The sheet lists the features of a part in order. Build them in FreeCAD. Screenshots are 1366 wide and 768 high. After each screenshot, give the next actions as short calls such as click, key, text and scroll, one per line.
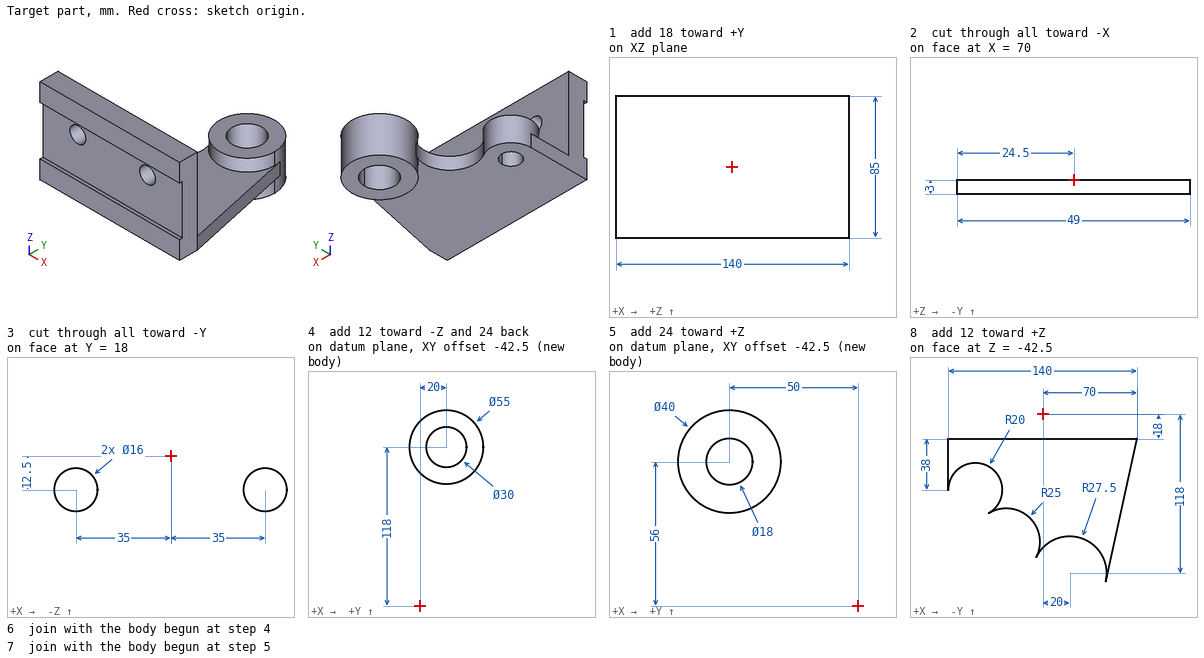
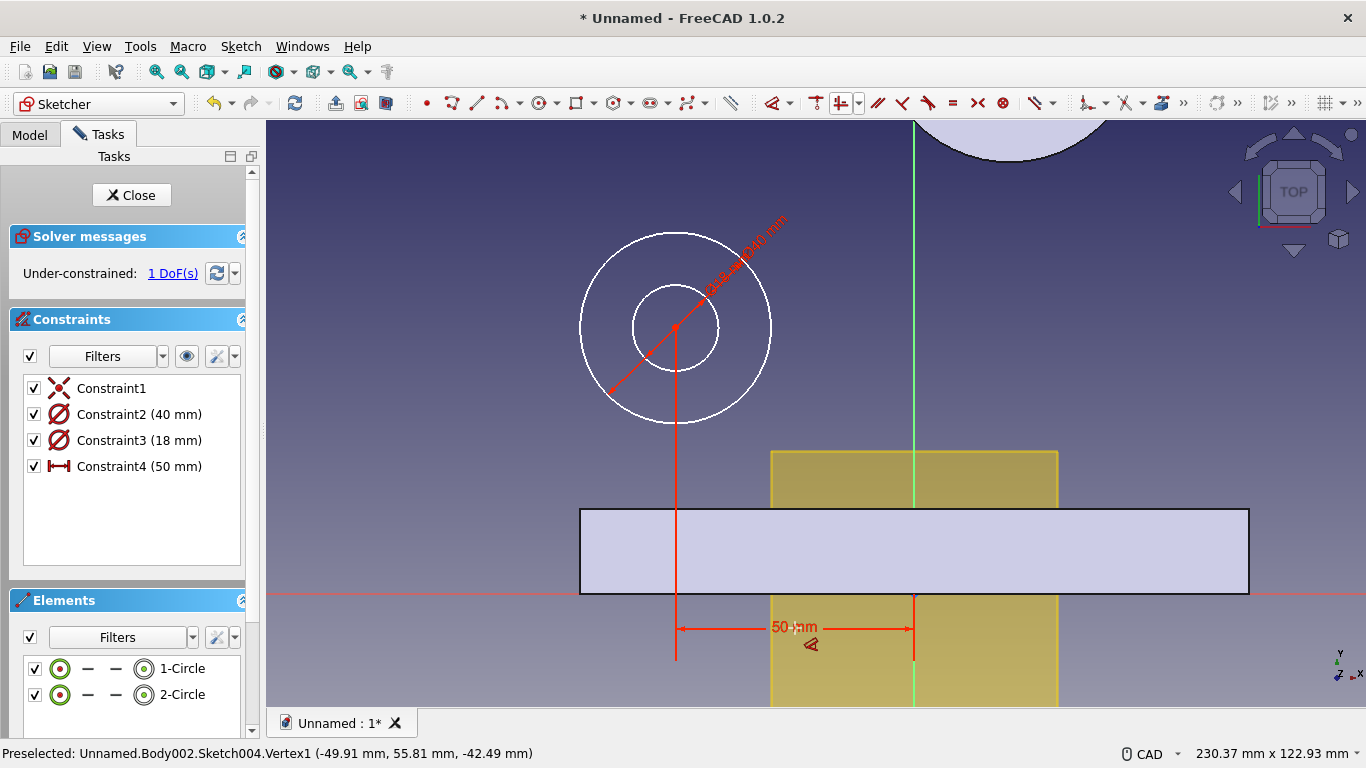
click(676, 328)
click(948, 461)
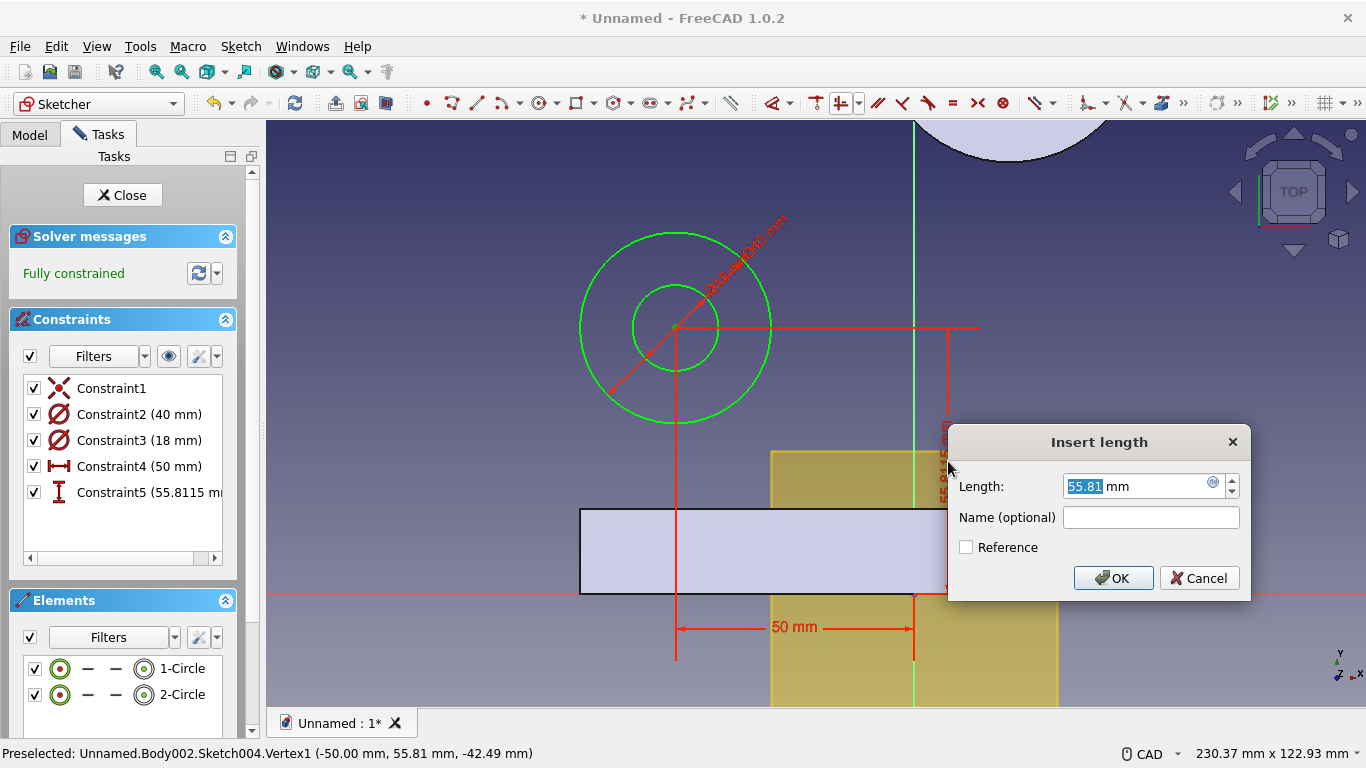
text(56)
key(Return)
key(Escape)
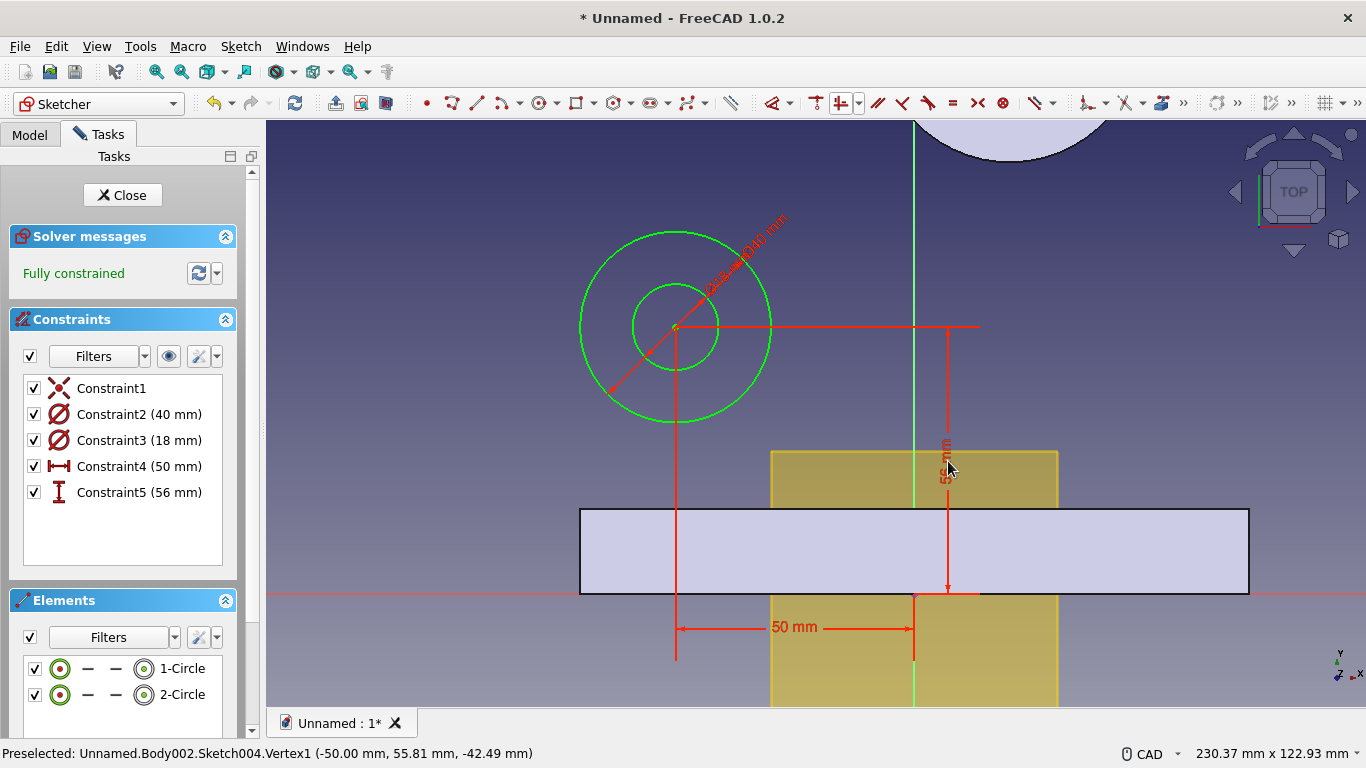
click(123, 195)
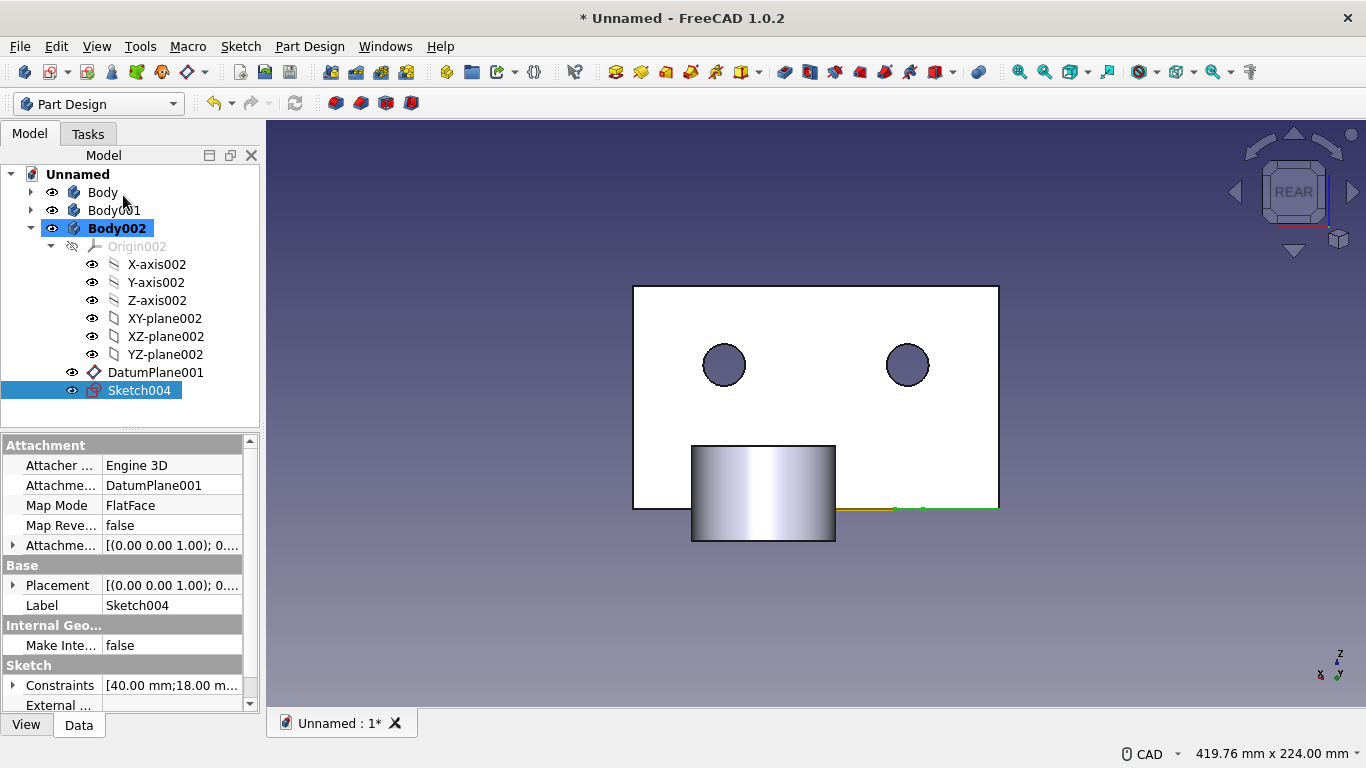
click(616, 72)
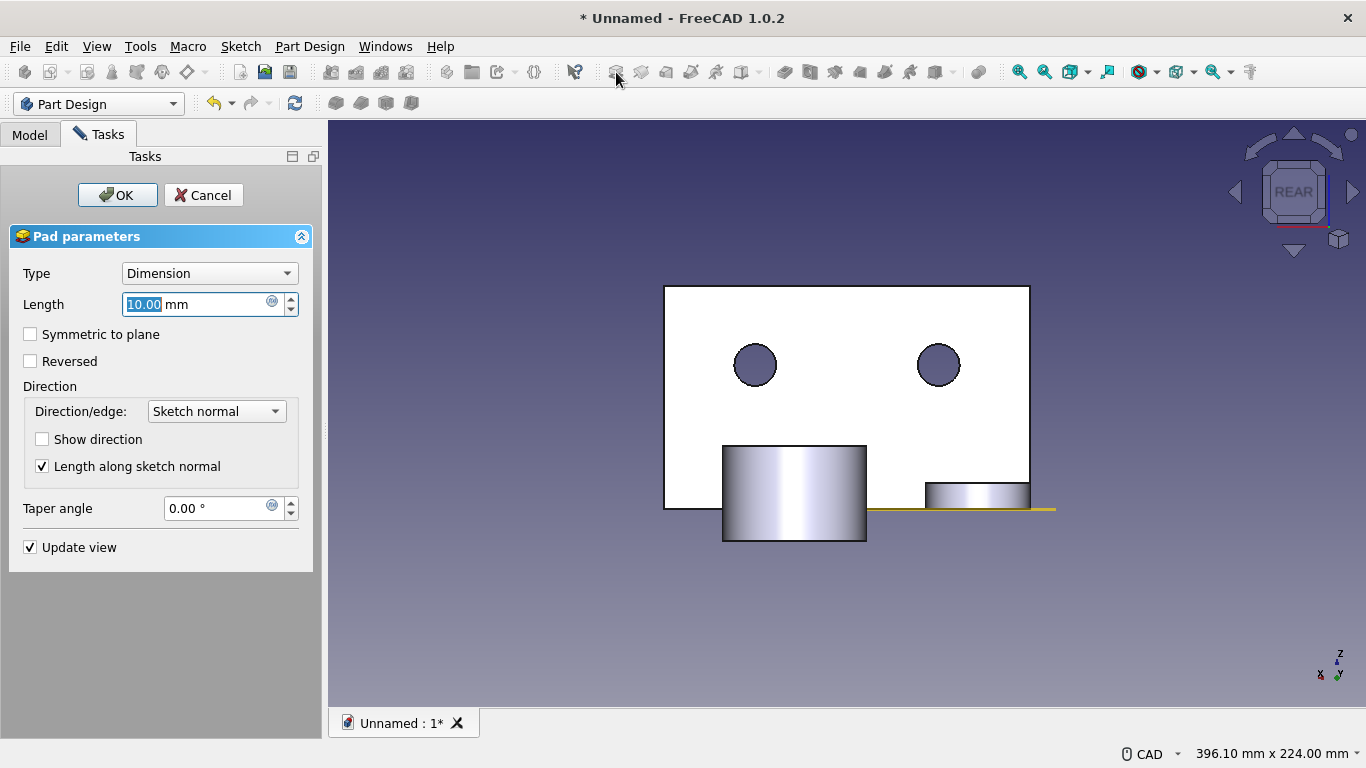
text(24)
key(Tab)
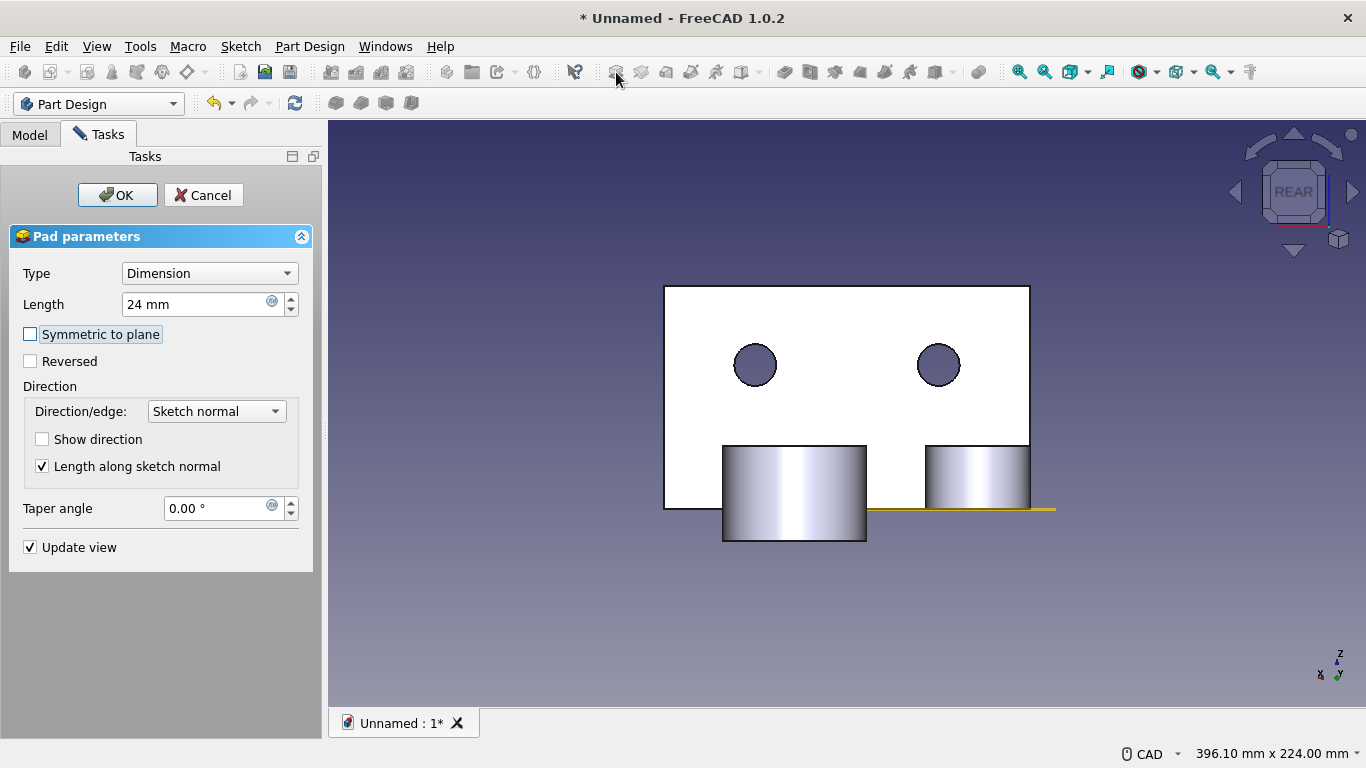
click(118, 195)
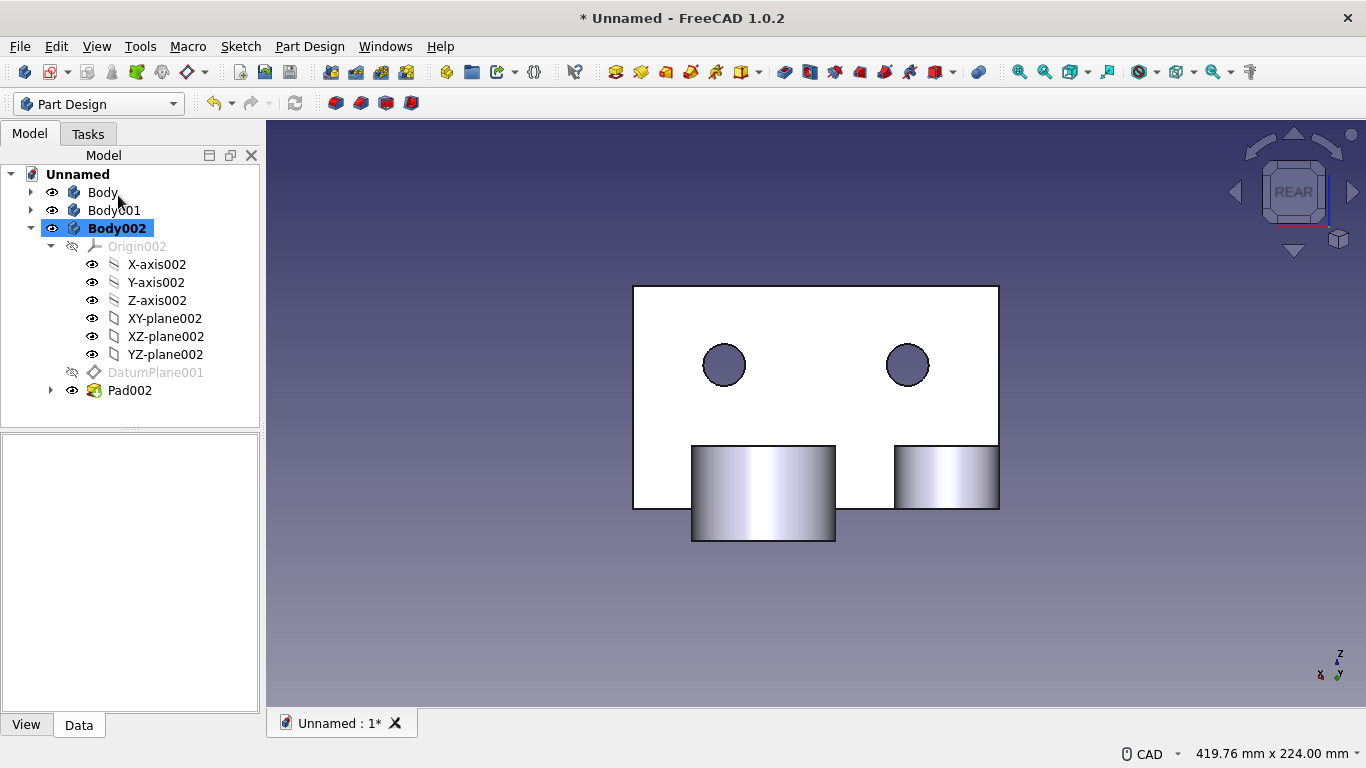
click(1020, 72)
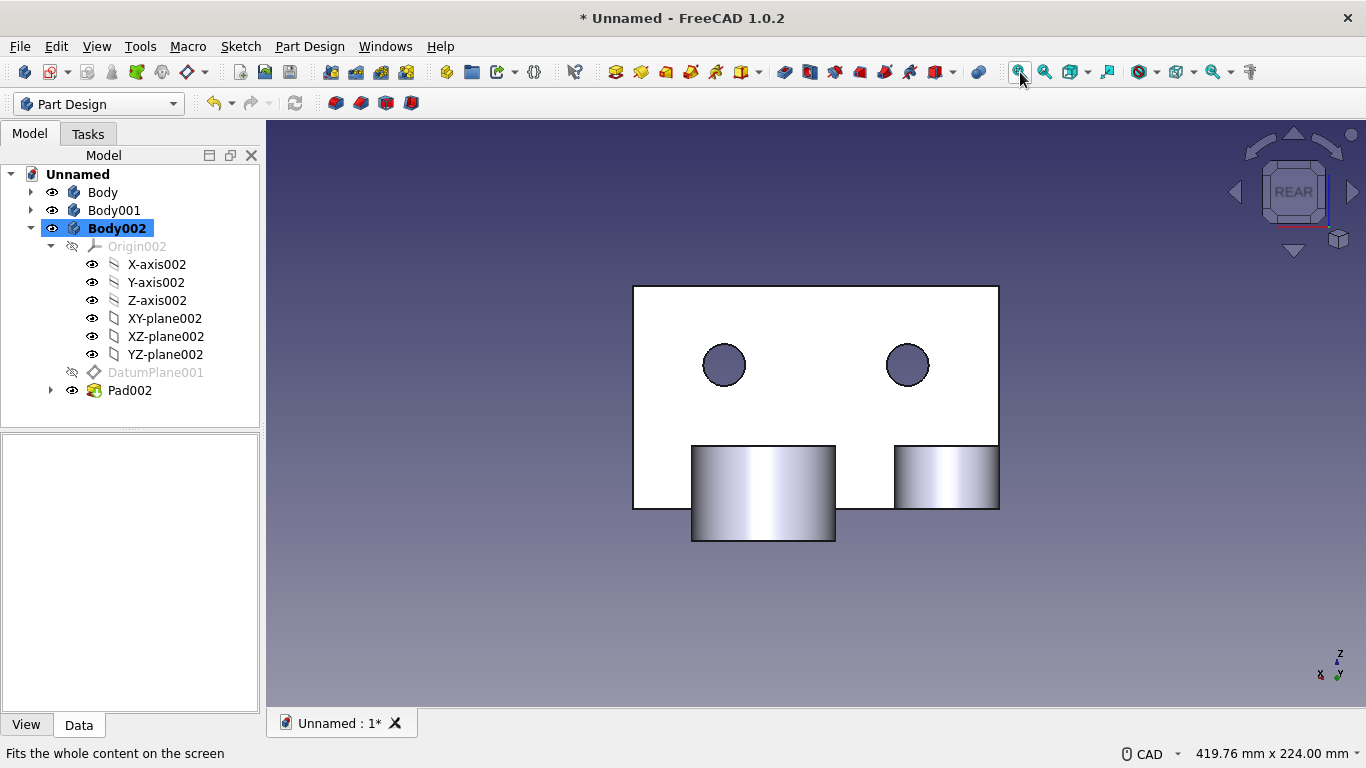
double_click(97, 192)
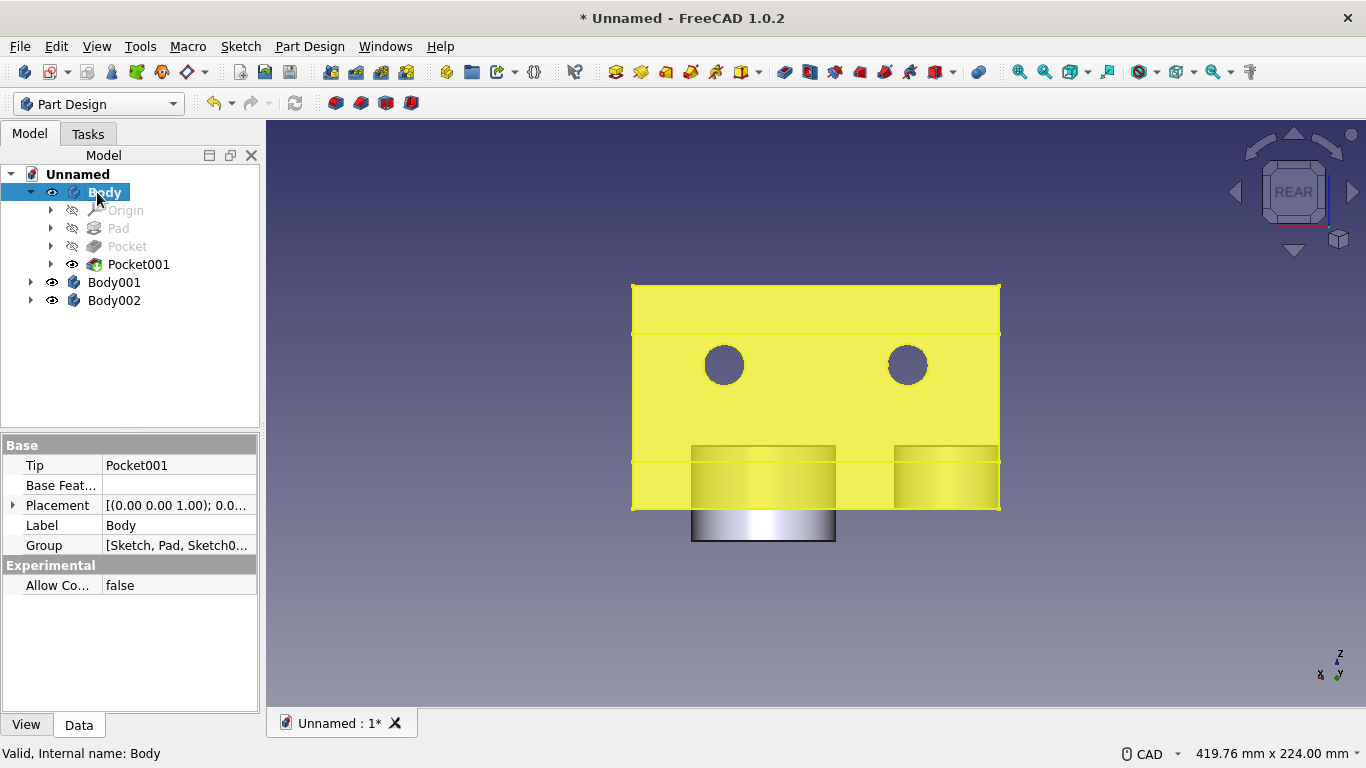
click(97, 192)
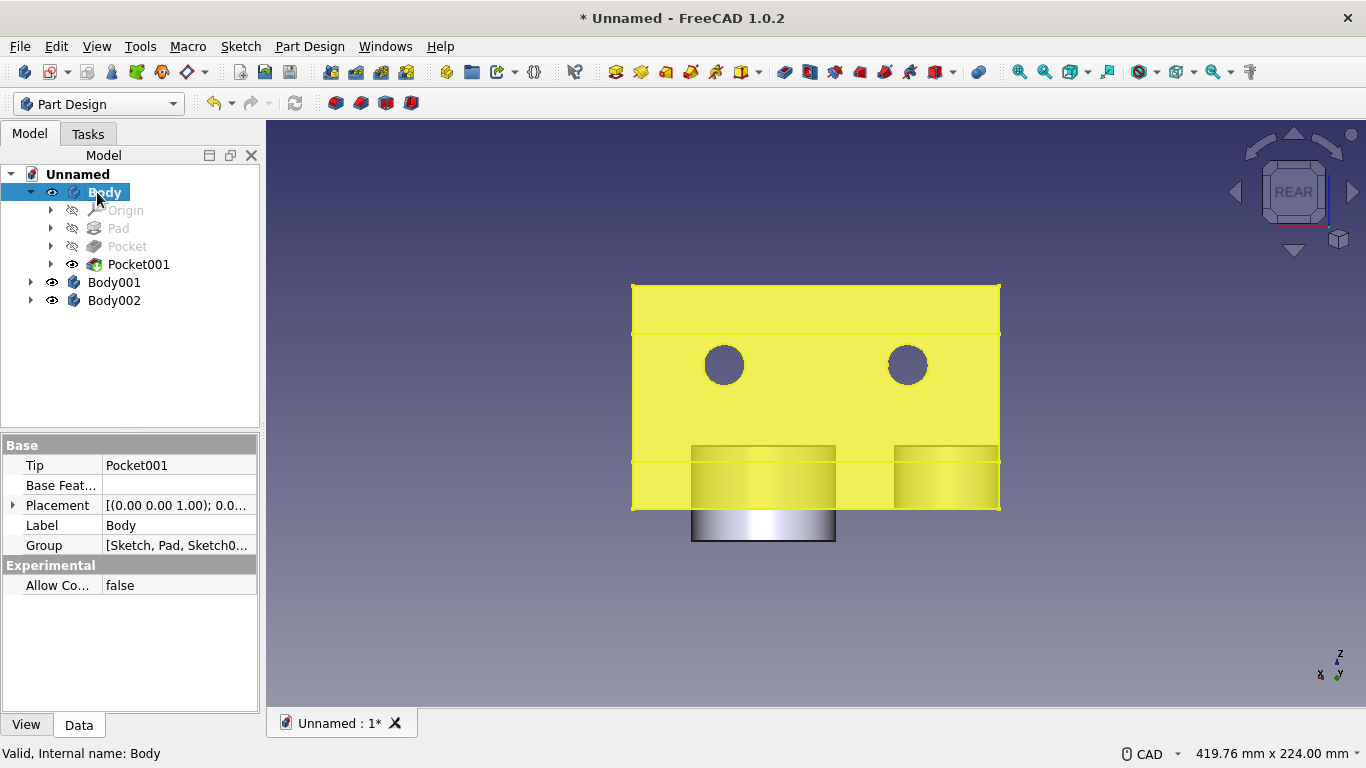
click(148, 585)